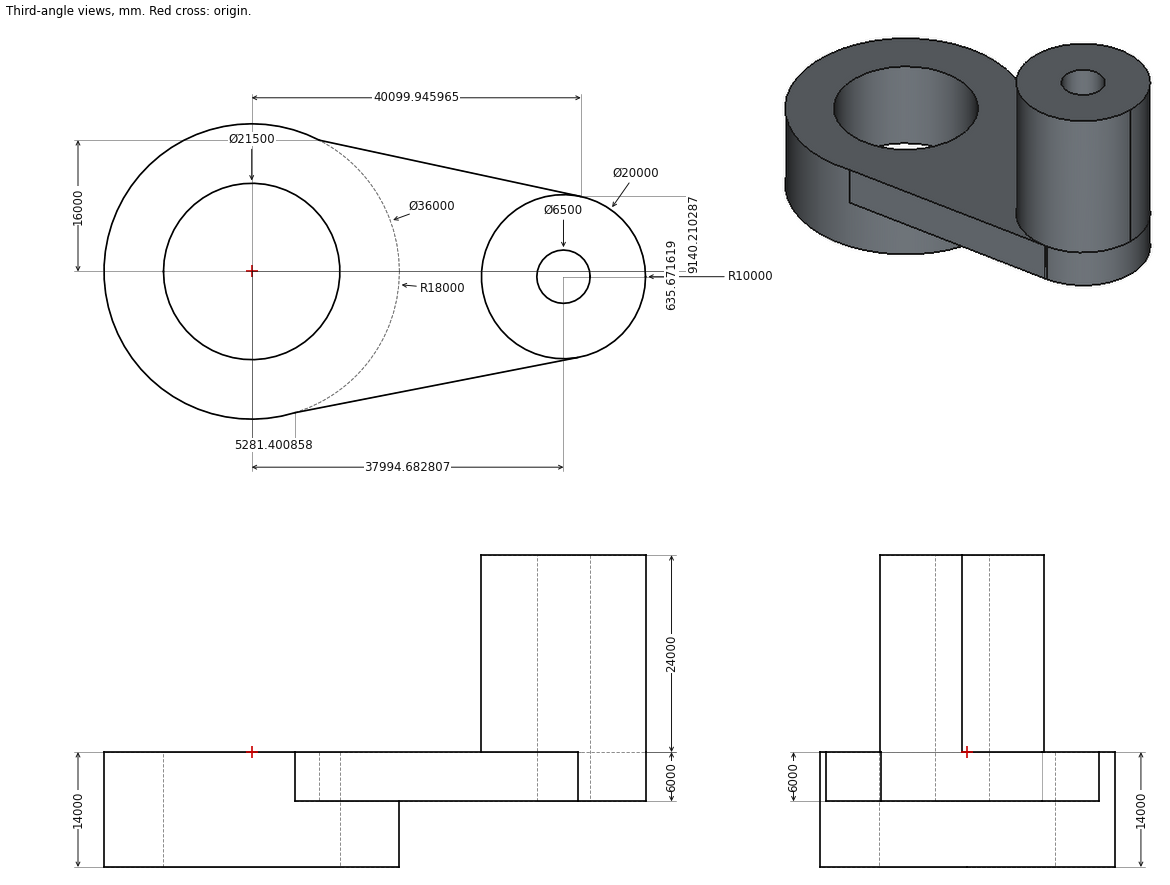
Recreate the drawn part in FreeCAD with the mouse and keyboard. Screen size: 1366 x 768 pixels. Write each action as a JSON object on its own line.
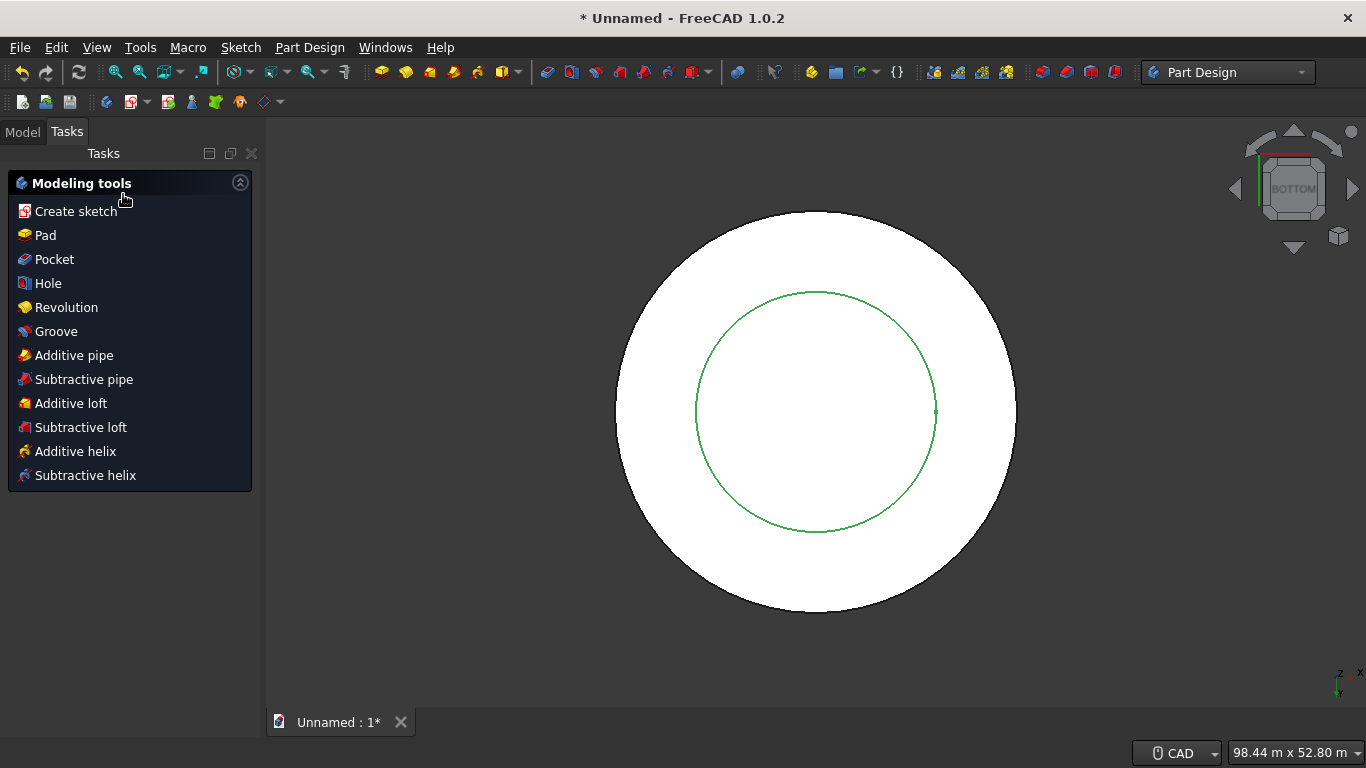
{"action": "left_click", "coordinate": [548, 72]}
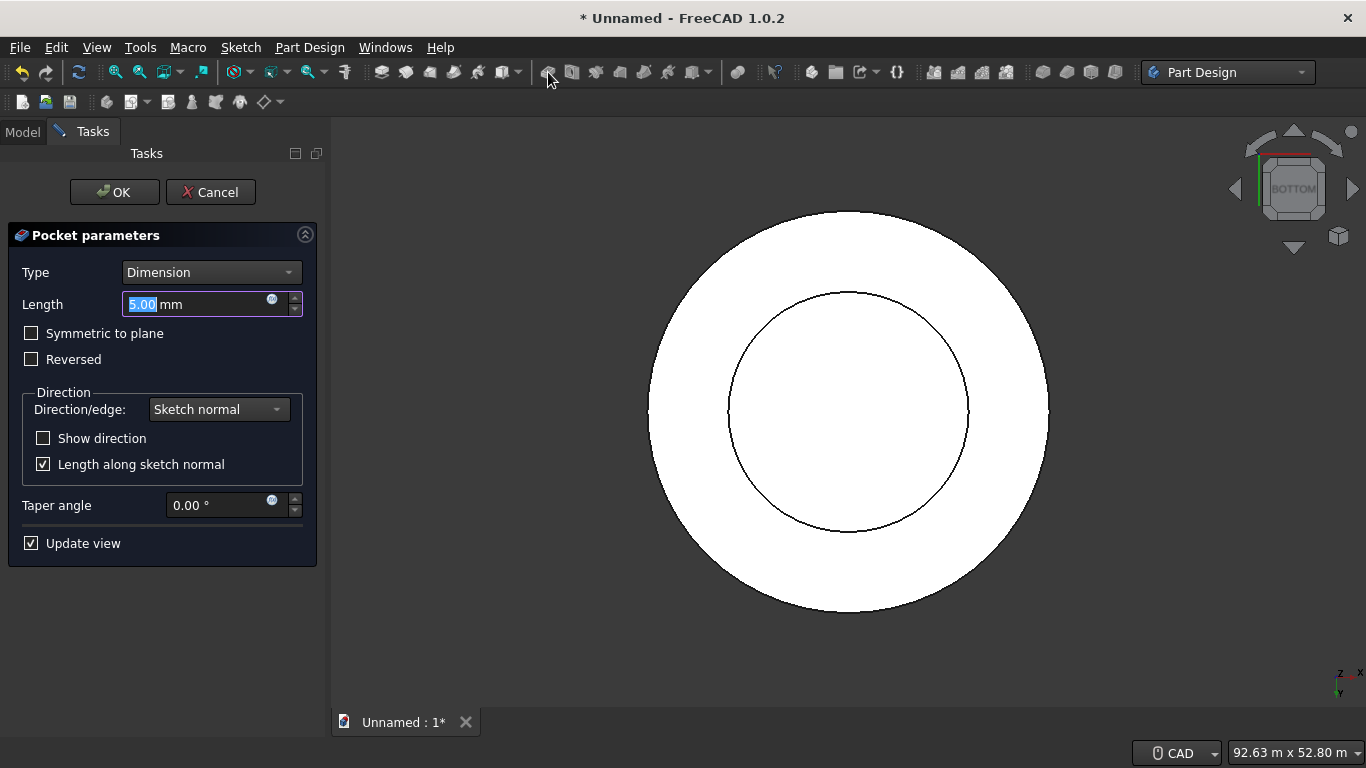
{"action": "type", "text": "14000"}
{"action": "key", "text": "Tab"}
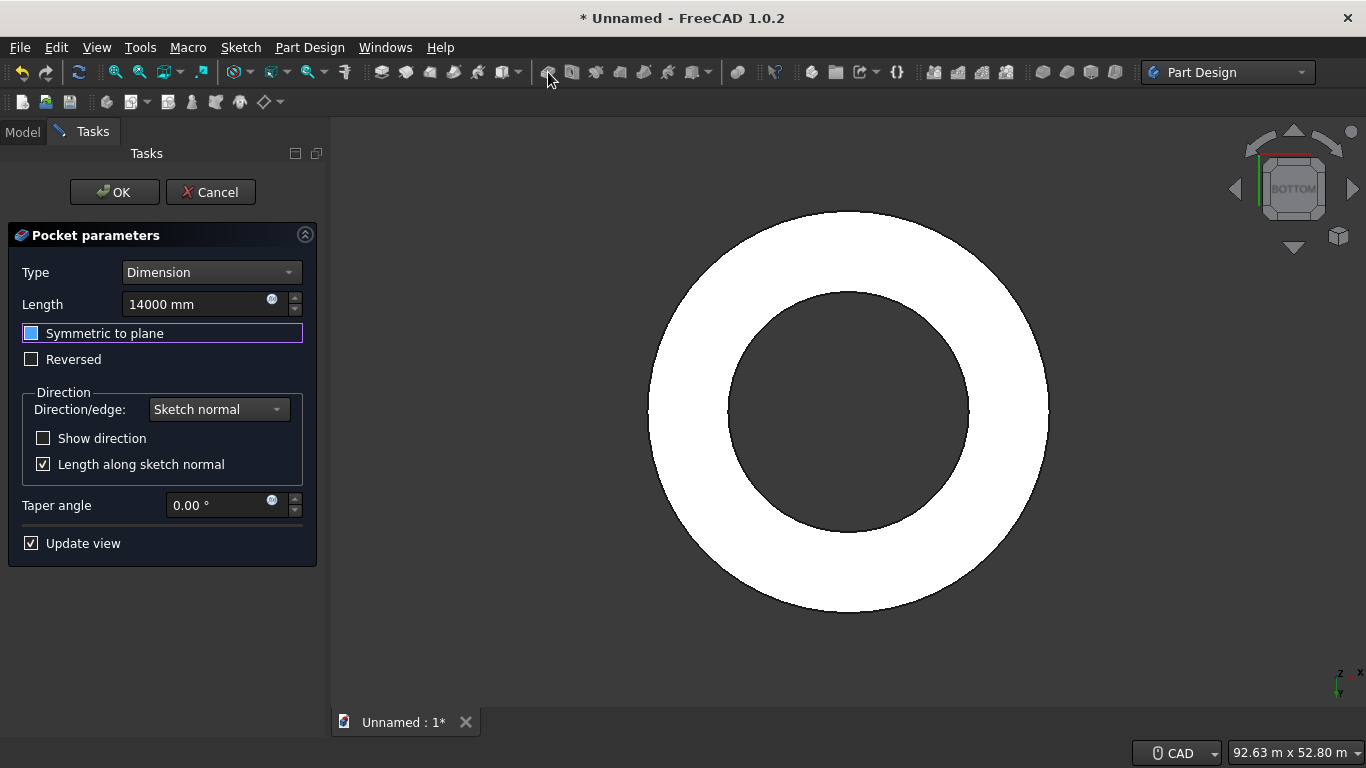
{"action": "left_click", "coordinate": [115, 192]}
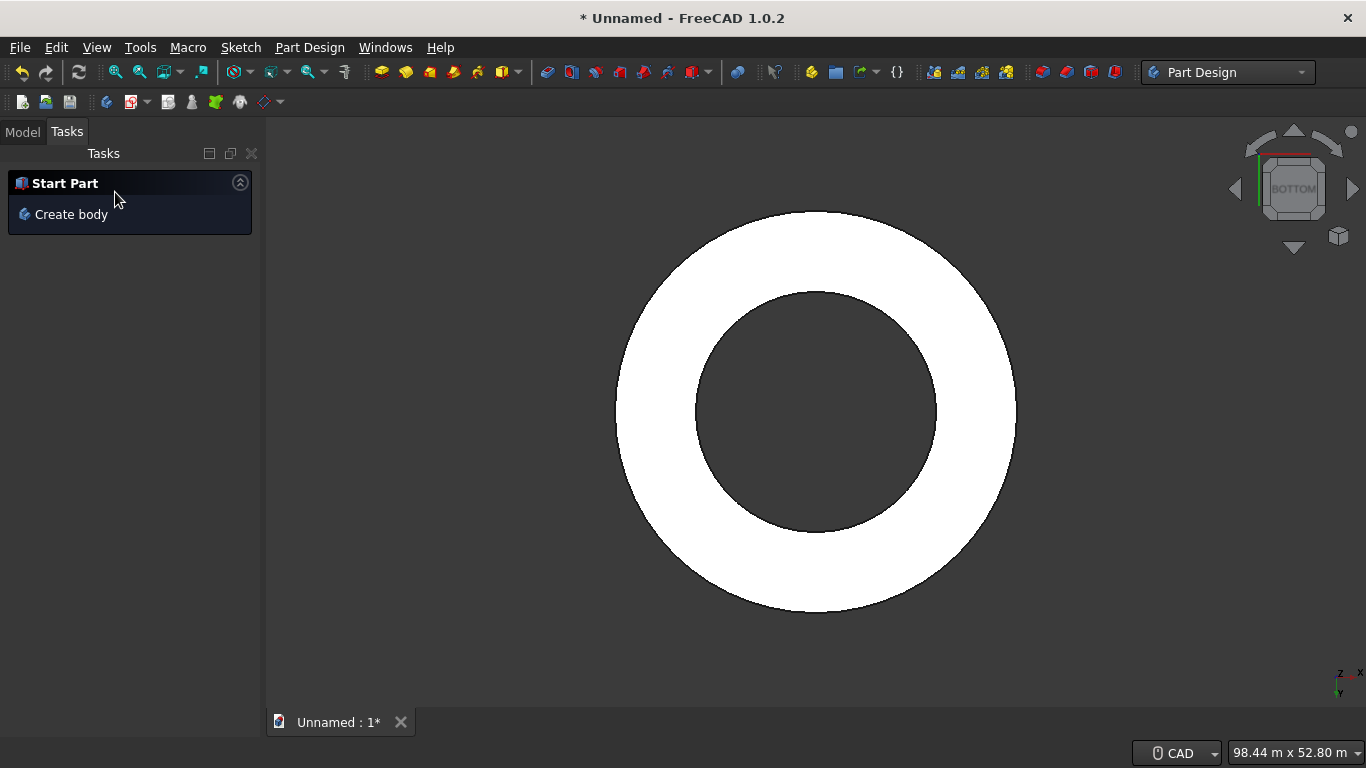
{"action": "left_click", "coordinate": [132, 102]}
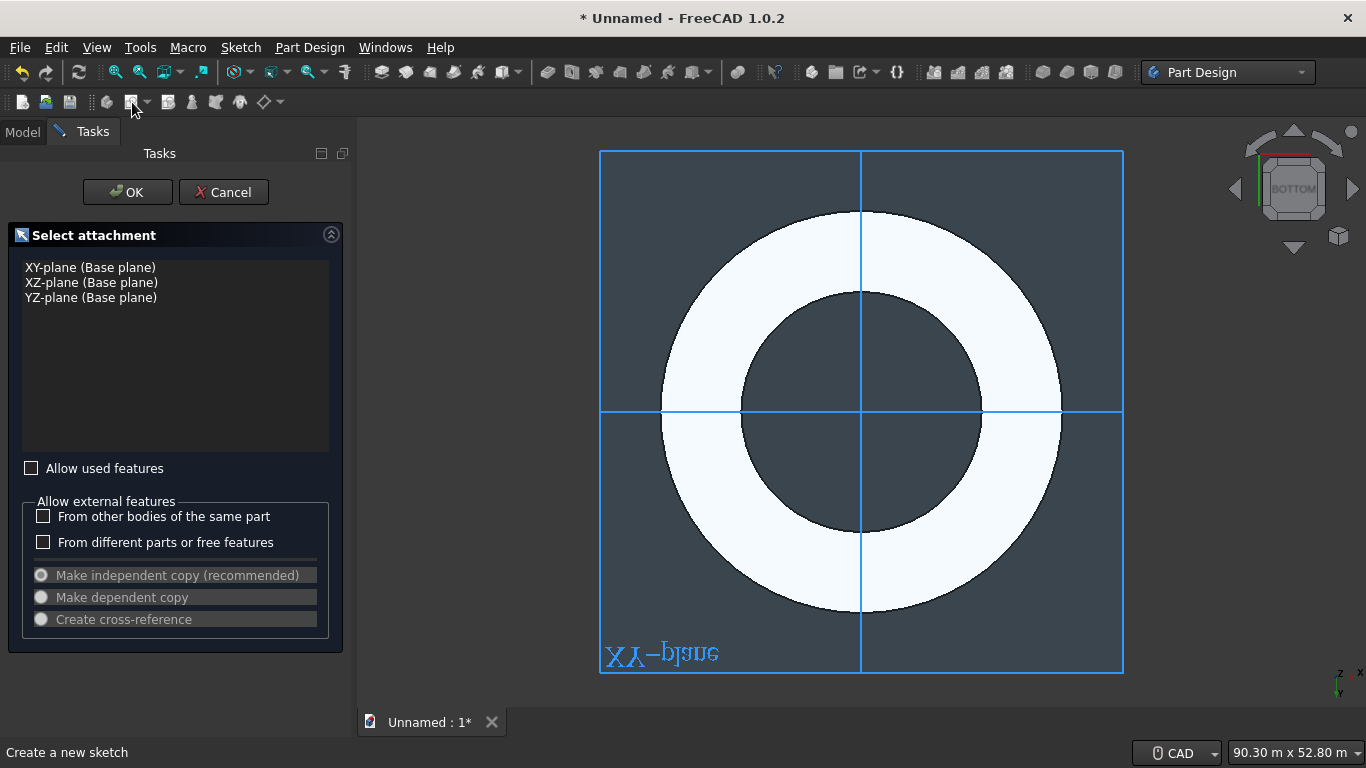
{"action": "left_click", "coordinate": [82, 268]}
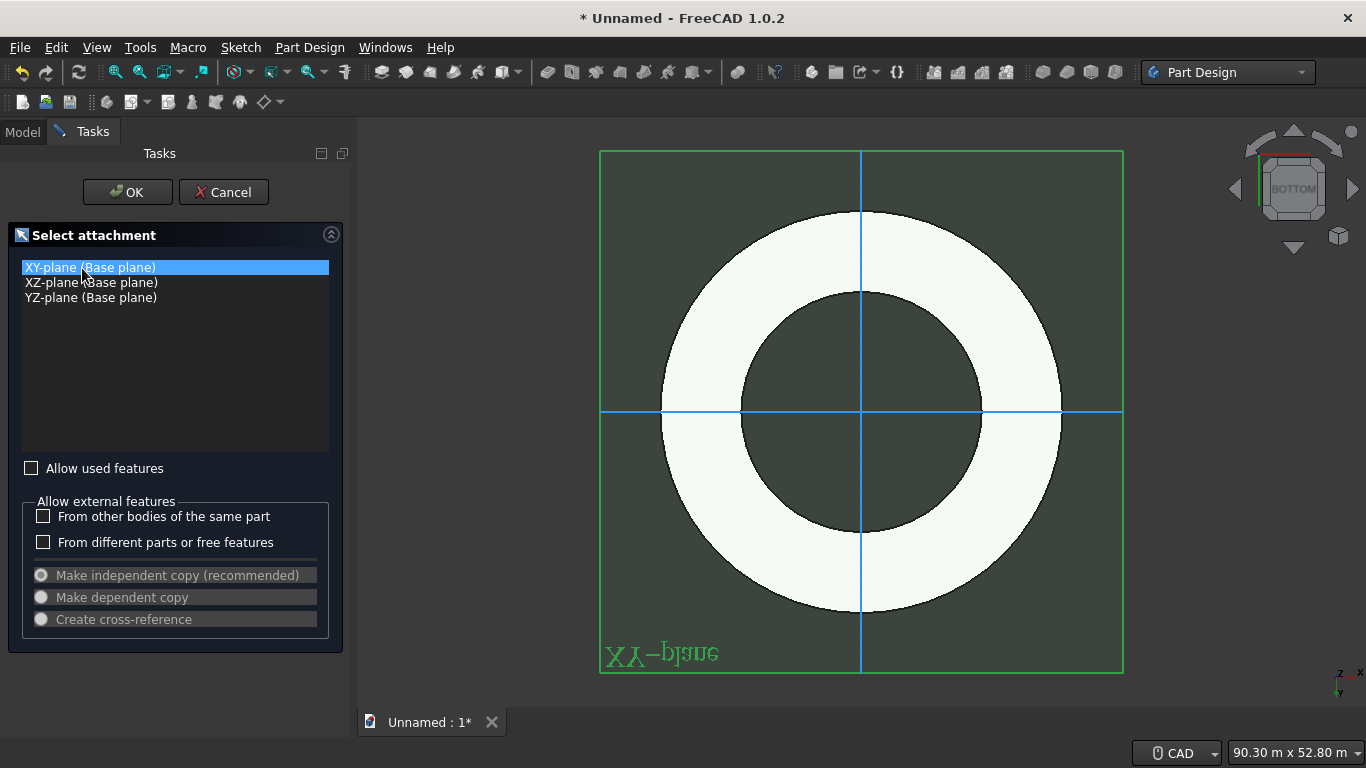
{"action": "left_click", "coordinate": [128, 192]}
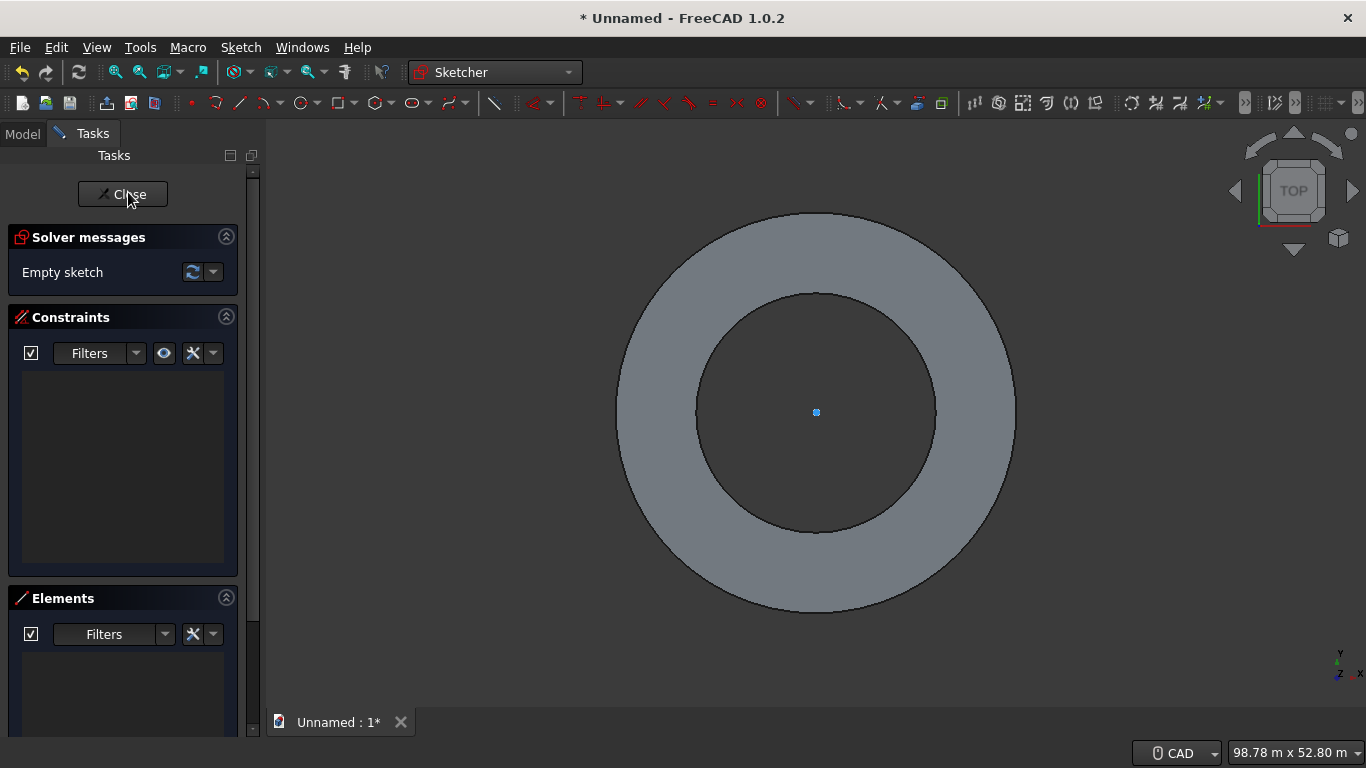
{"action": "scroll", "coordinate": [294, 383], "scroll_direction": "down", "scroll_amount": 1}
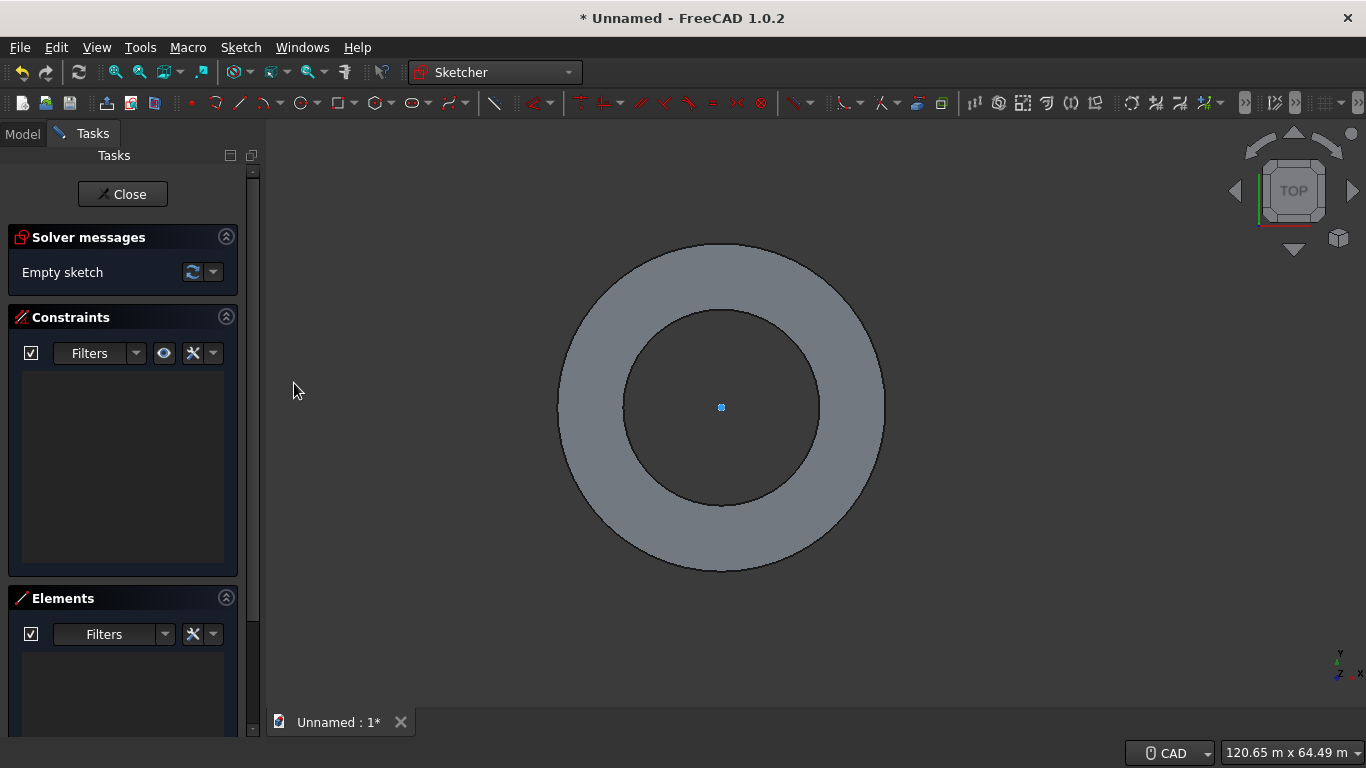
{"action": "left_click", "coordinate": [240, 104]}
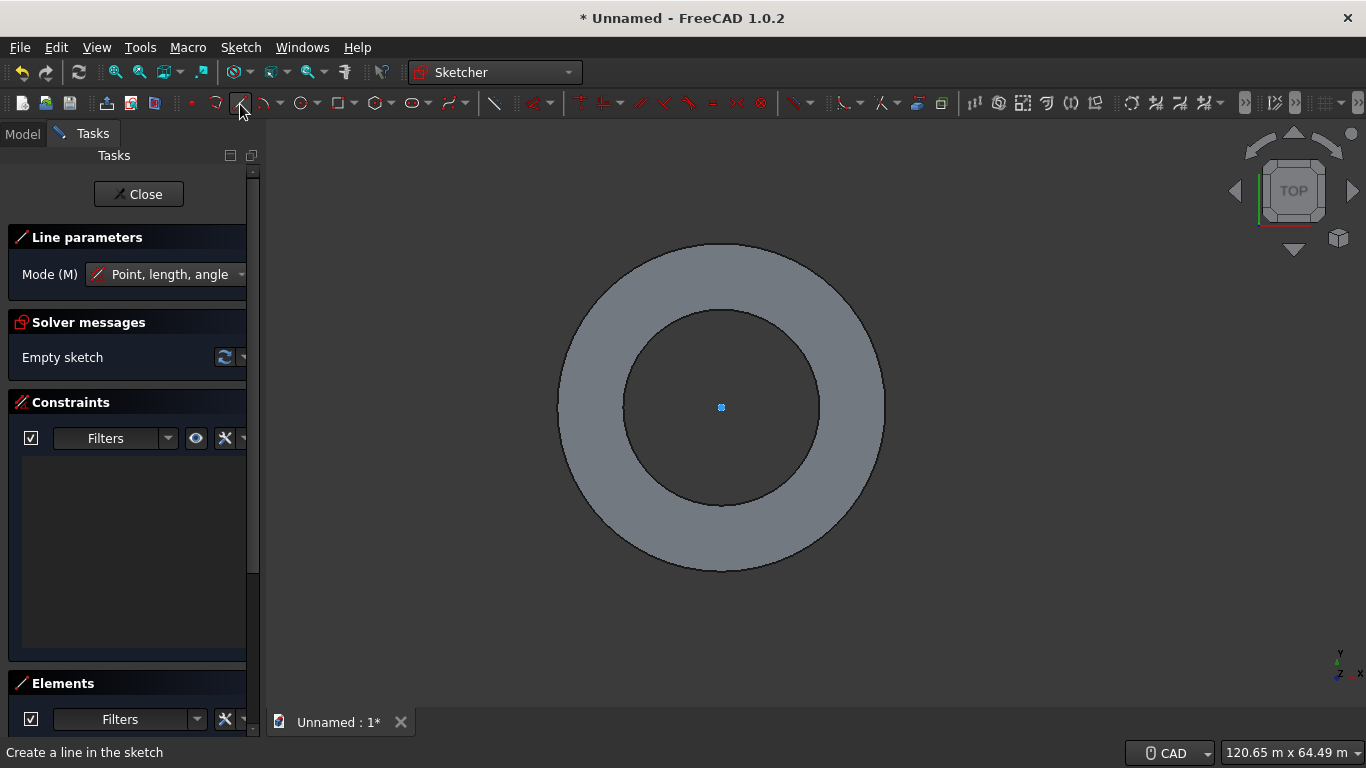
{"action": "left_click", "coordinate": [1087, 324]}
{"action": "left_click", "coordinate": [797, 262]}